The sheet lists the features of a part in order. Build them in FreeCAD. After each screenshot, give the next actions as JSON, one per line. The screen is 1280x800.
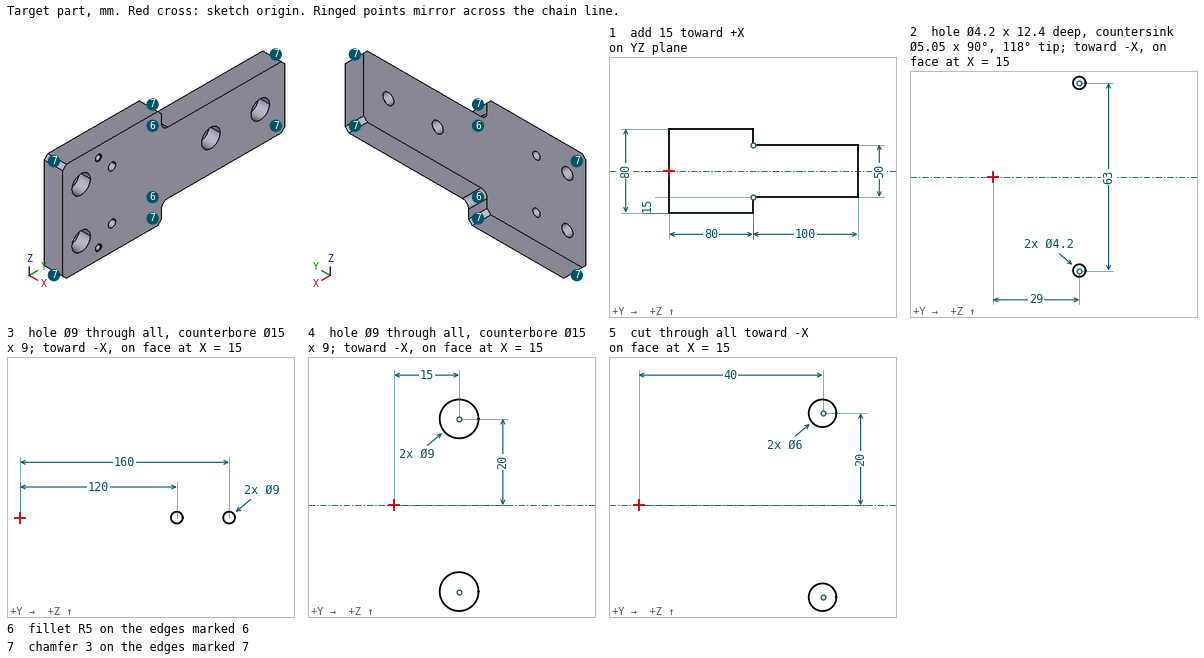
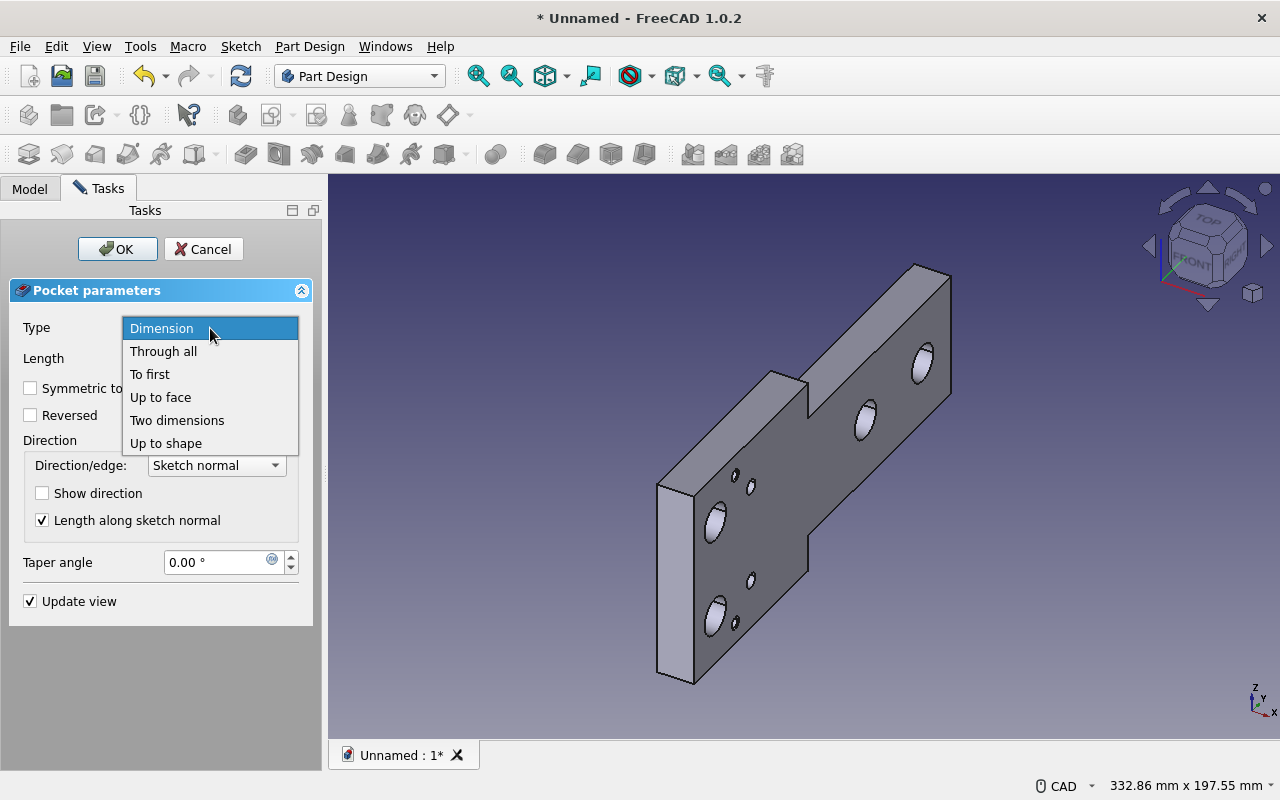
{"action": "left_click", "coordinate": [208, 352]}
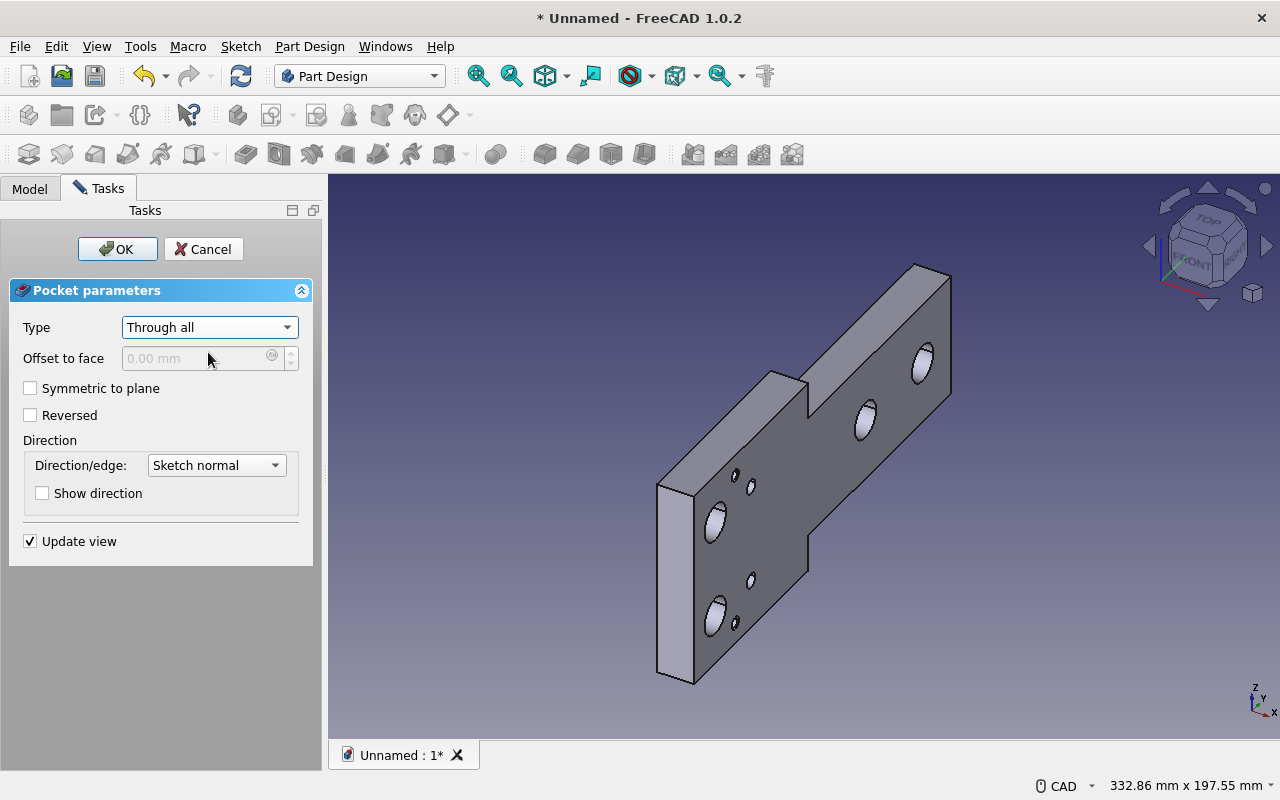
{"action": "left_click", "coordinate": [118, 249]}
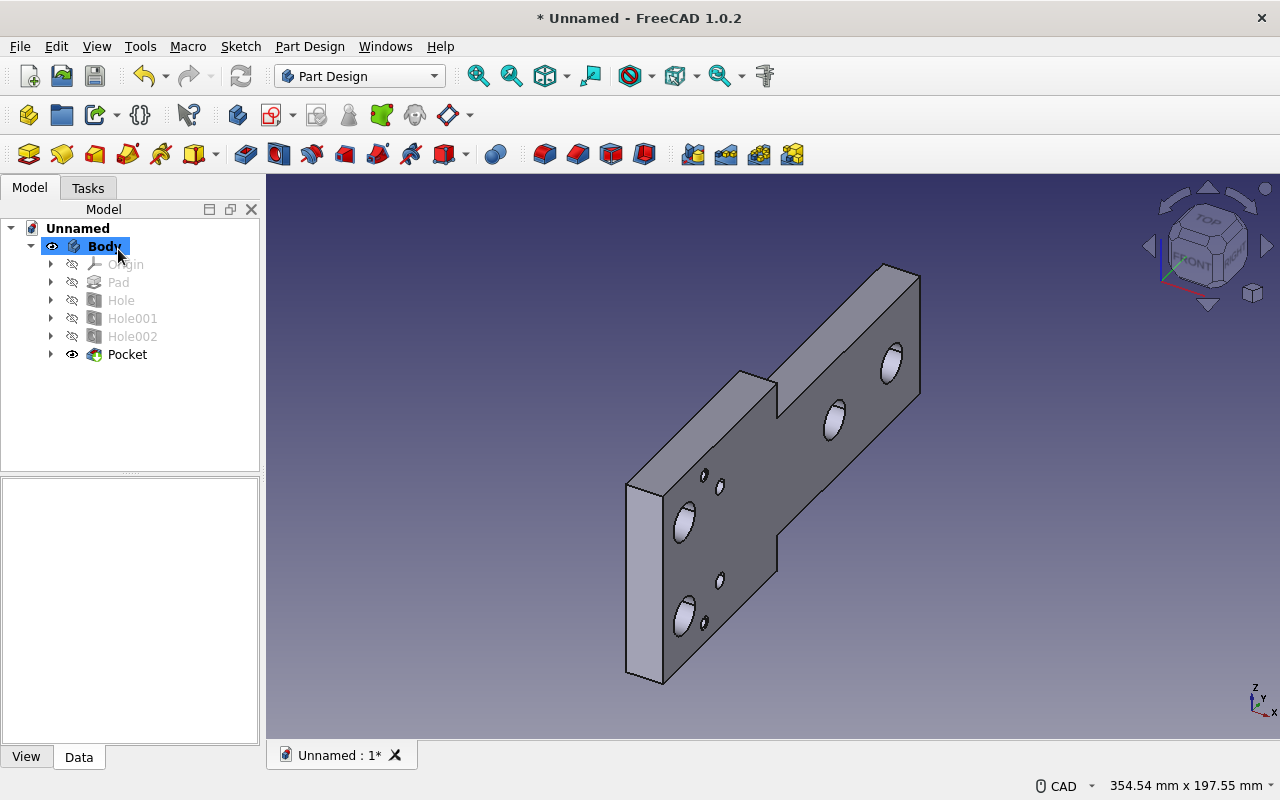
{"action": "key", "text": "0"}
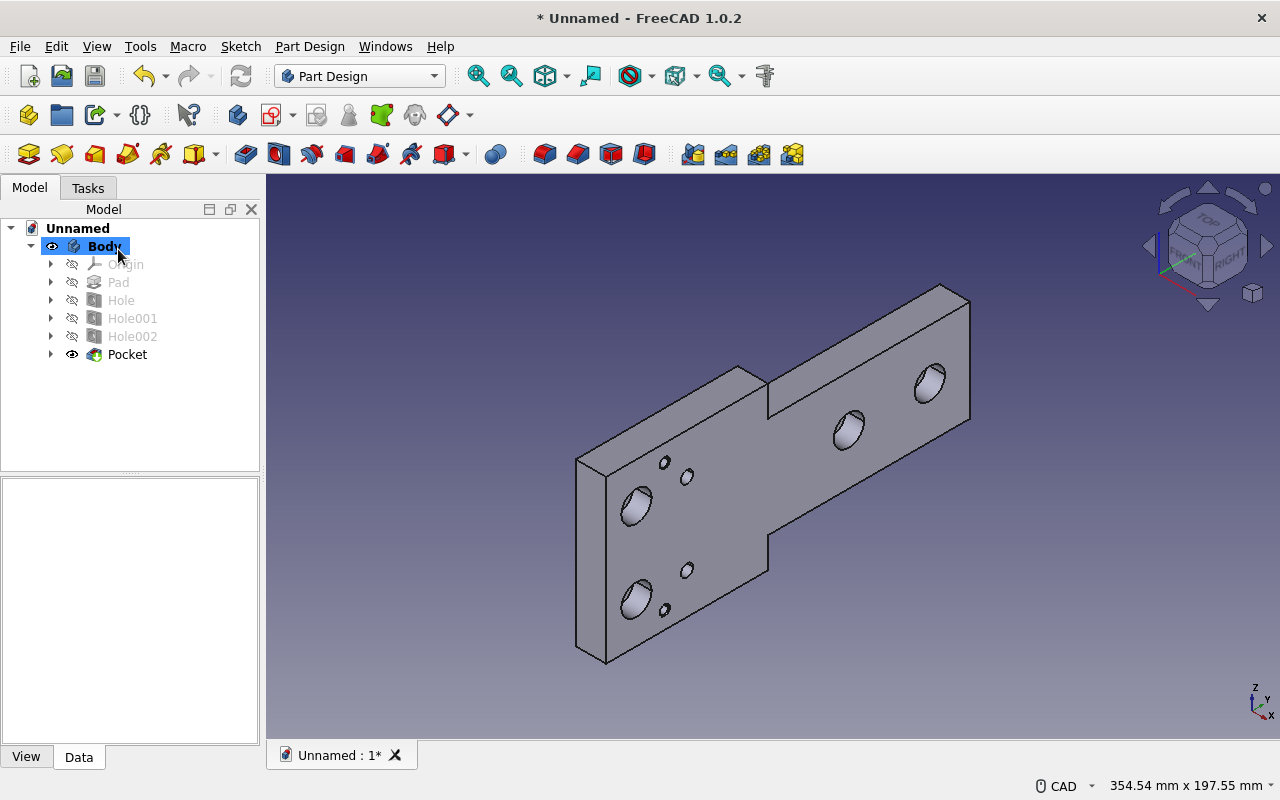
{"action": "key", "text": "2"}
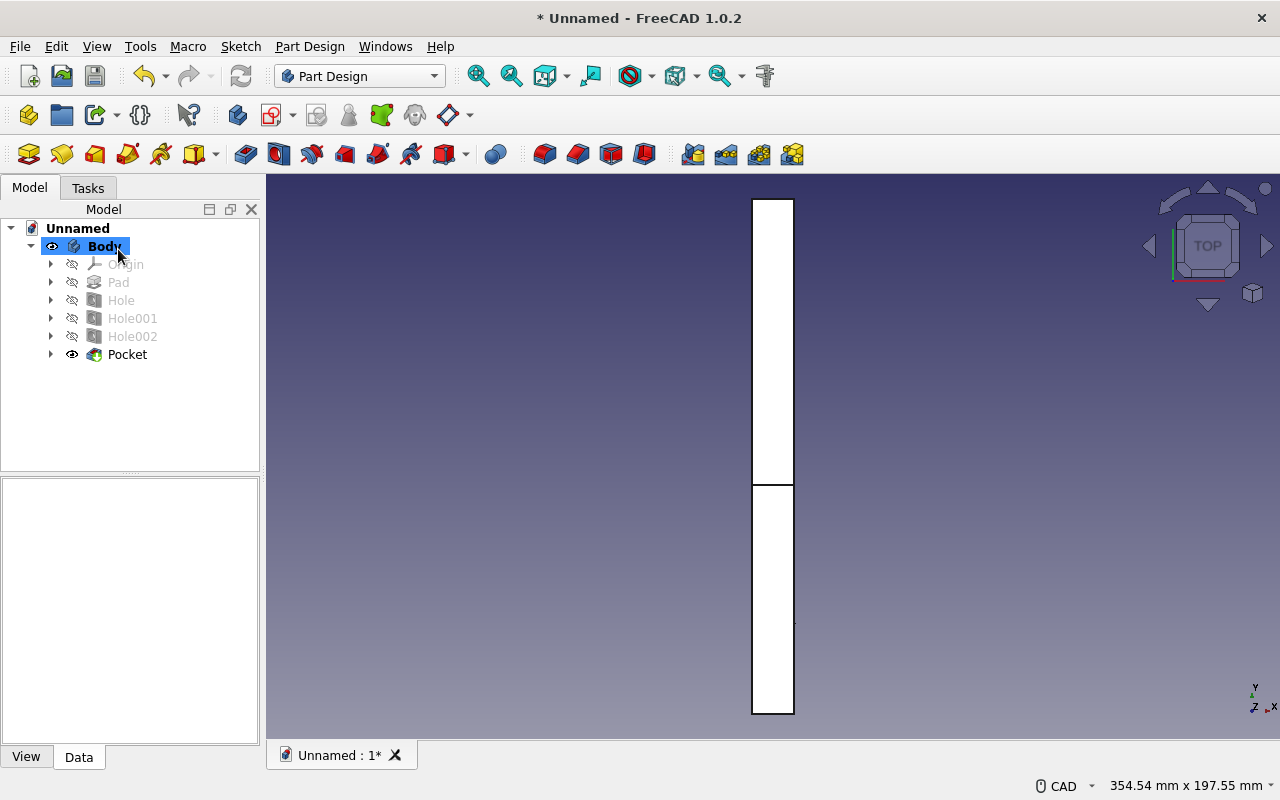
{"action": "key", "text": "1"}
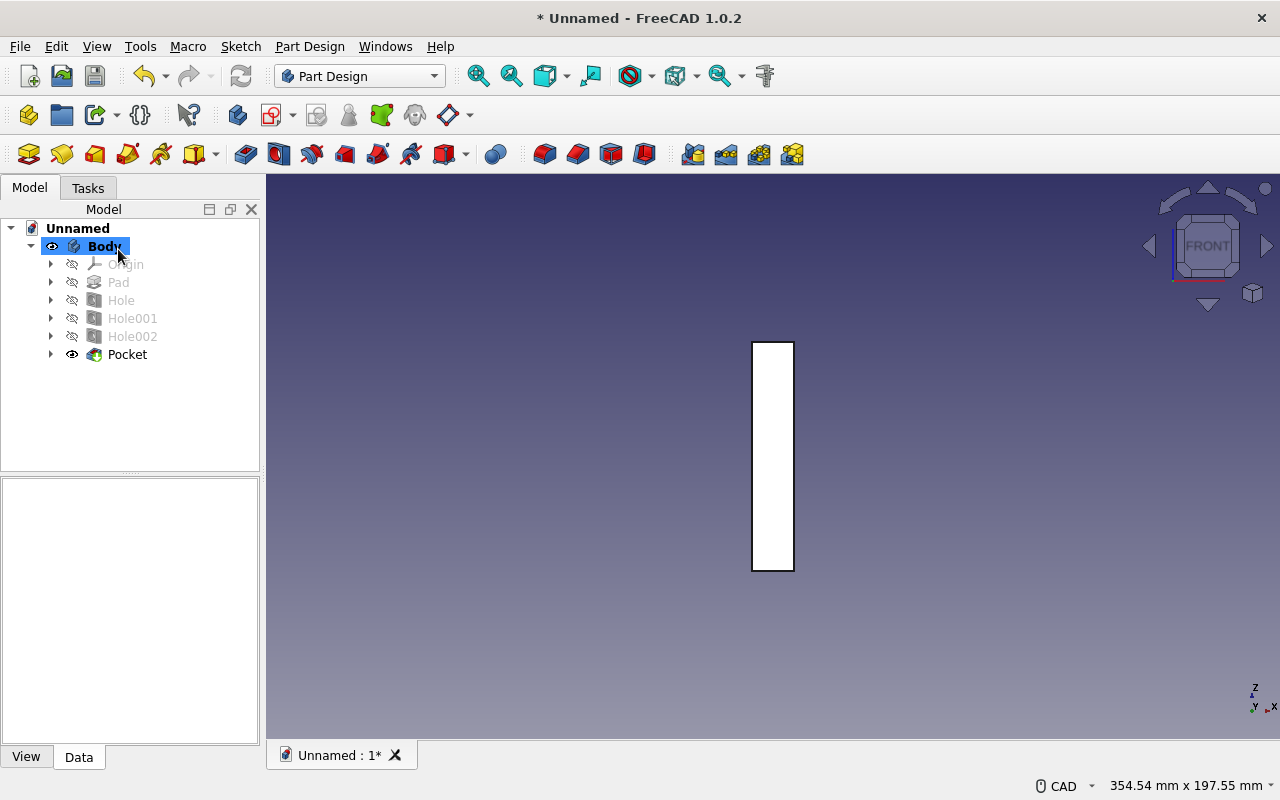
{"action": "left_click", "coordinate": [479, 76]}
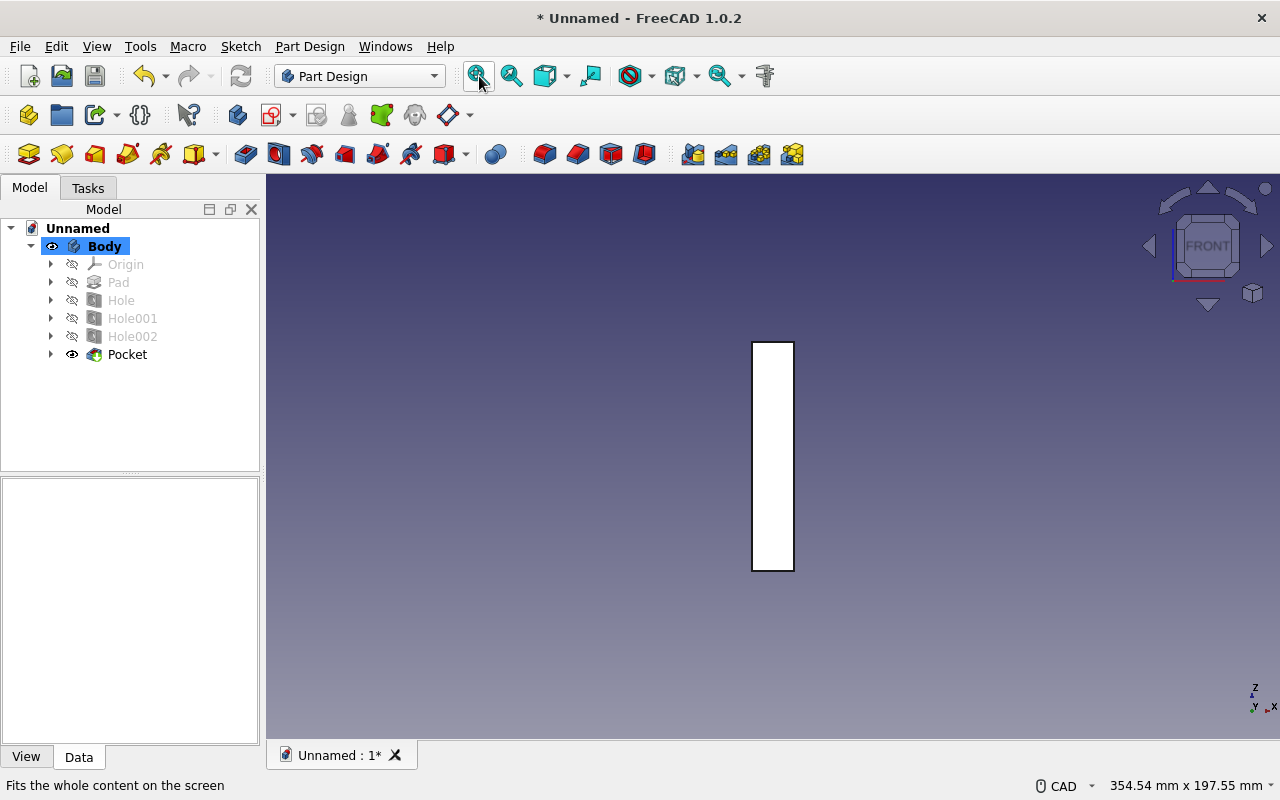
{"action": "key", "text": "3"}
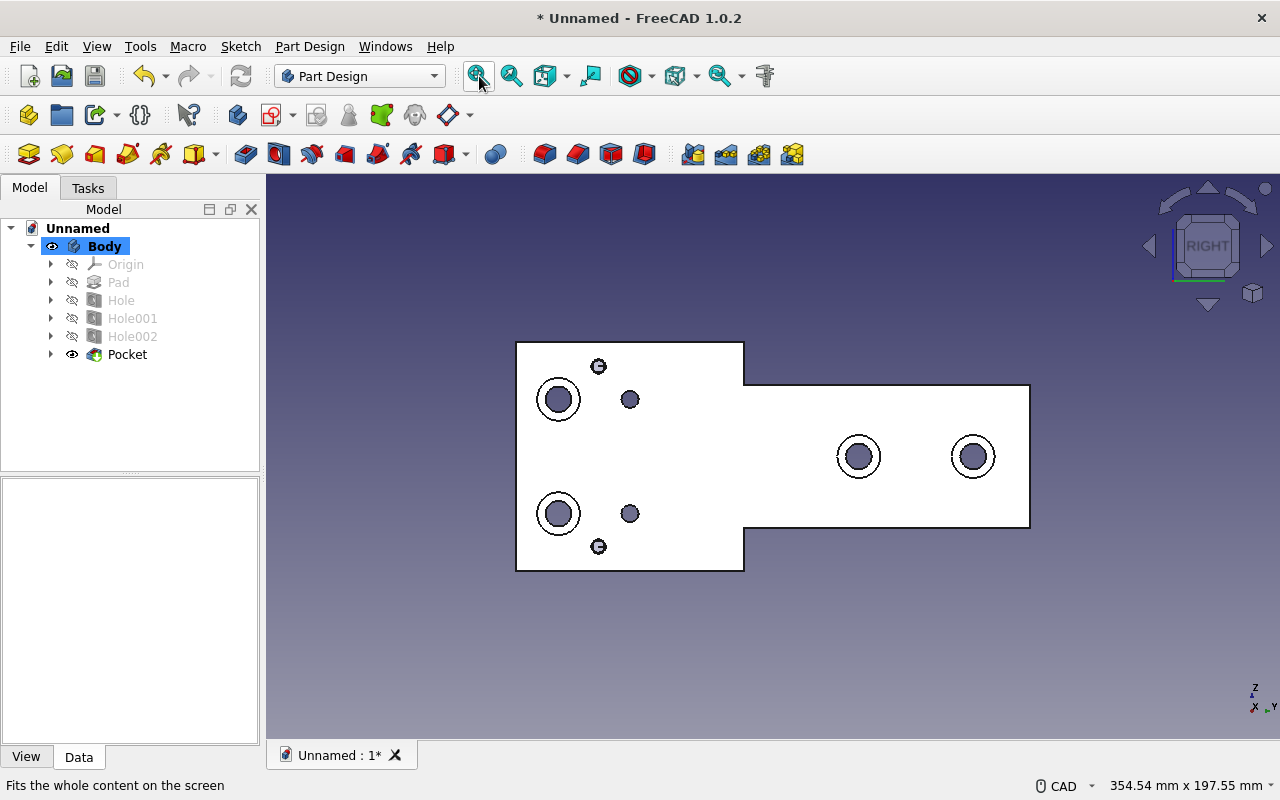
{"action": "key", "text": "5"}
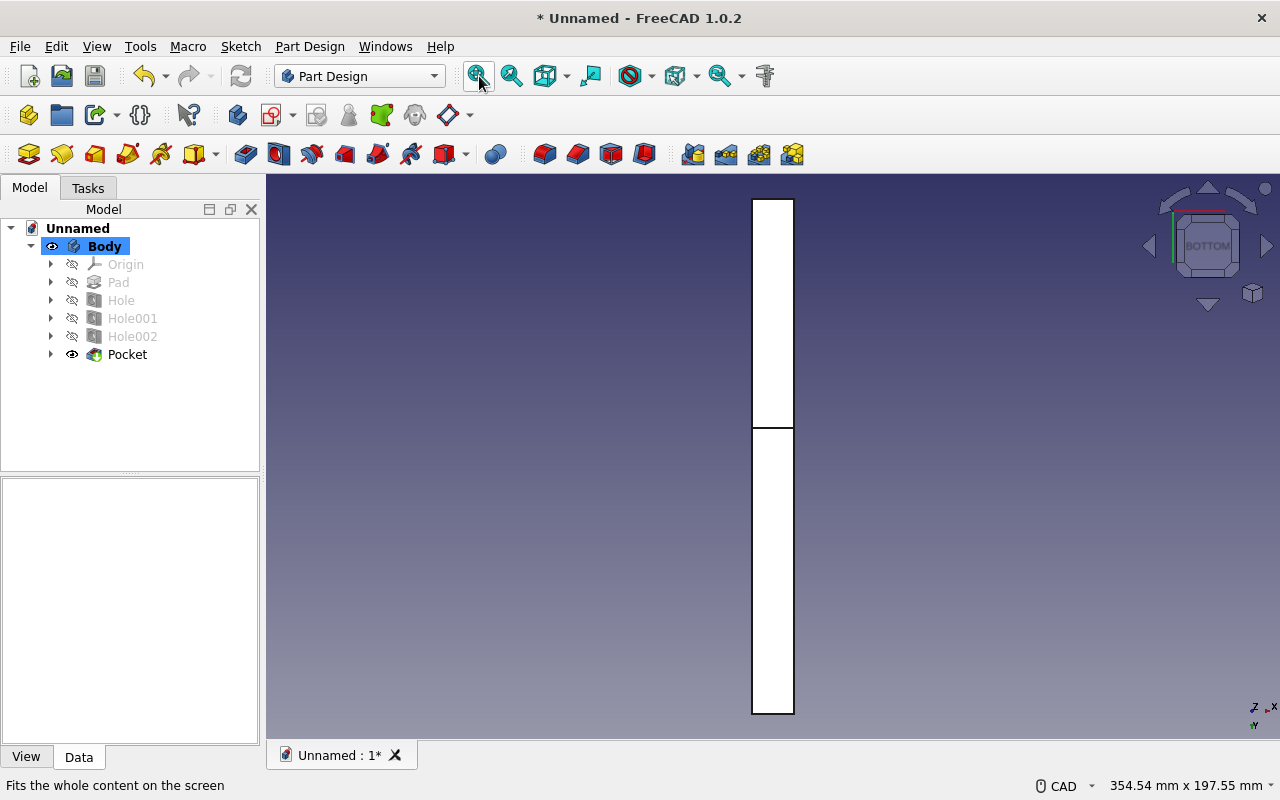
{"action": "key", "text": "4"}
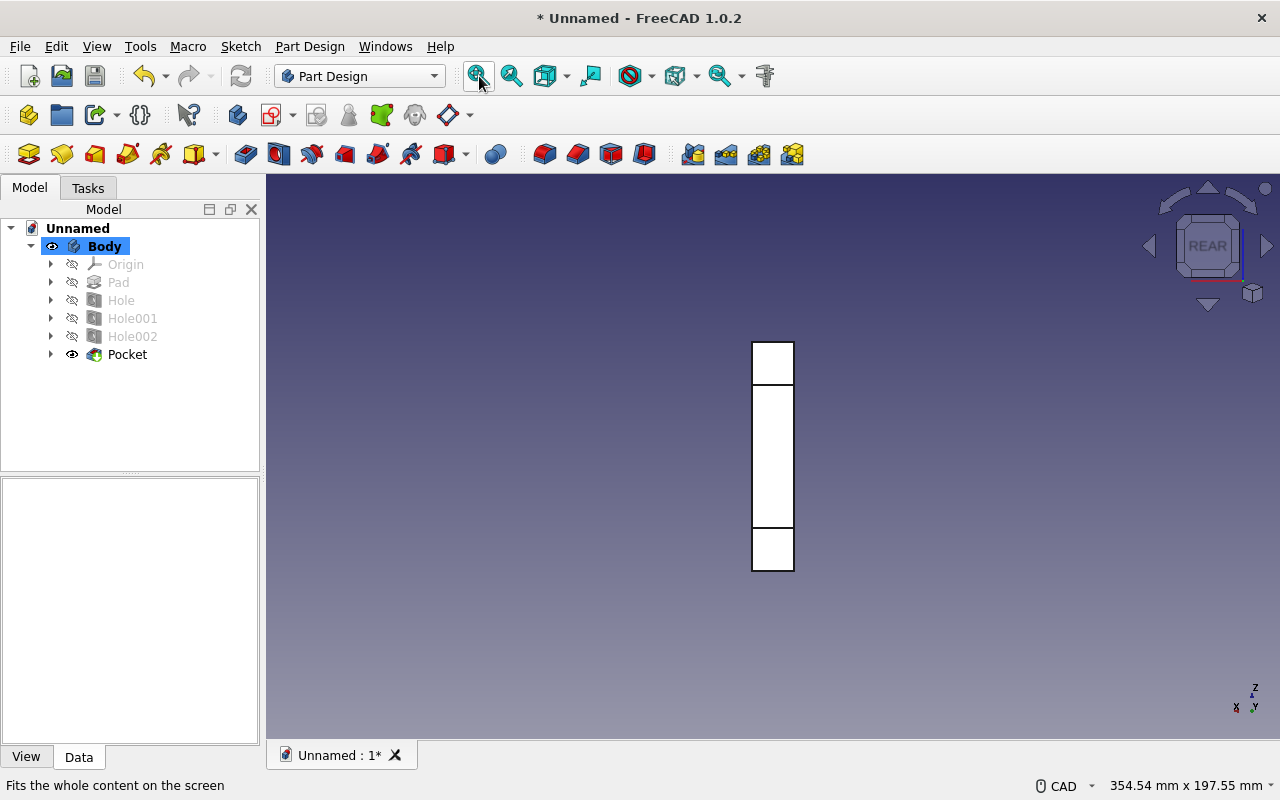
{"action": "key", "text": "v f"}